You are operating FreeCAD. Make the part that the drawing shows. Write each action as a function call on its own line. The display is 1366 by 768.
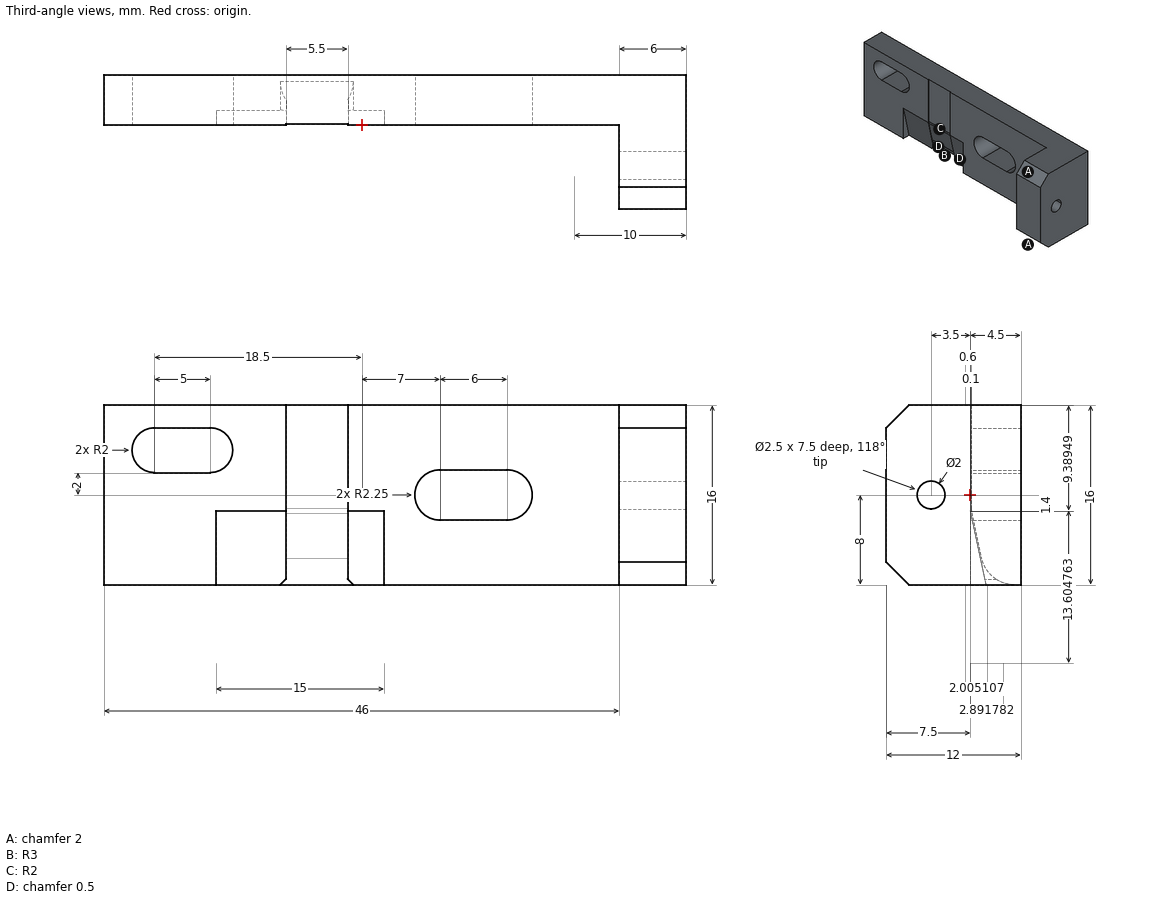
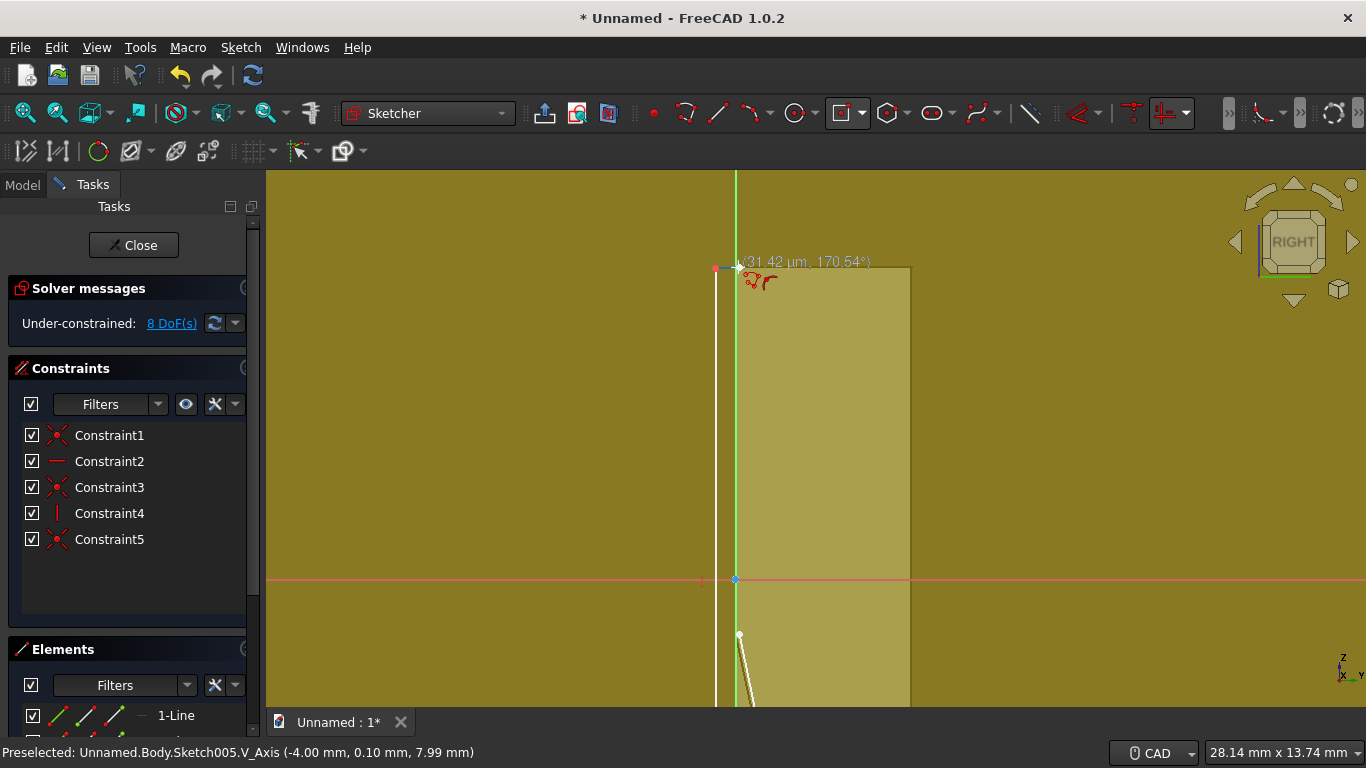
scroll(739, 469, up, 11)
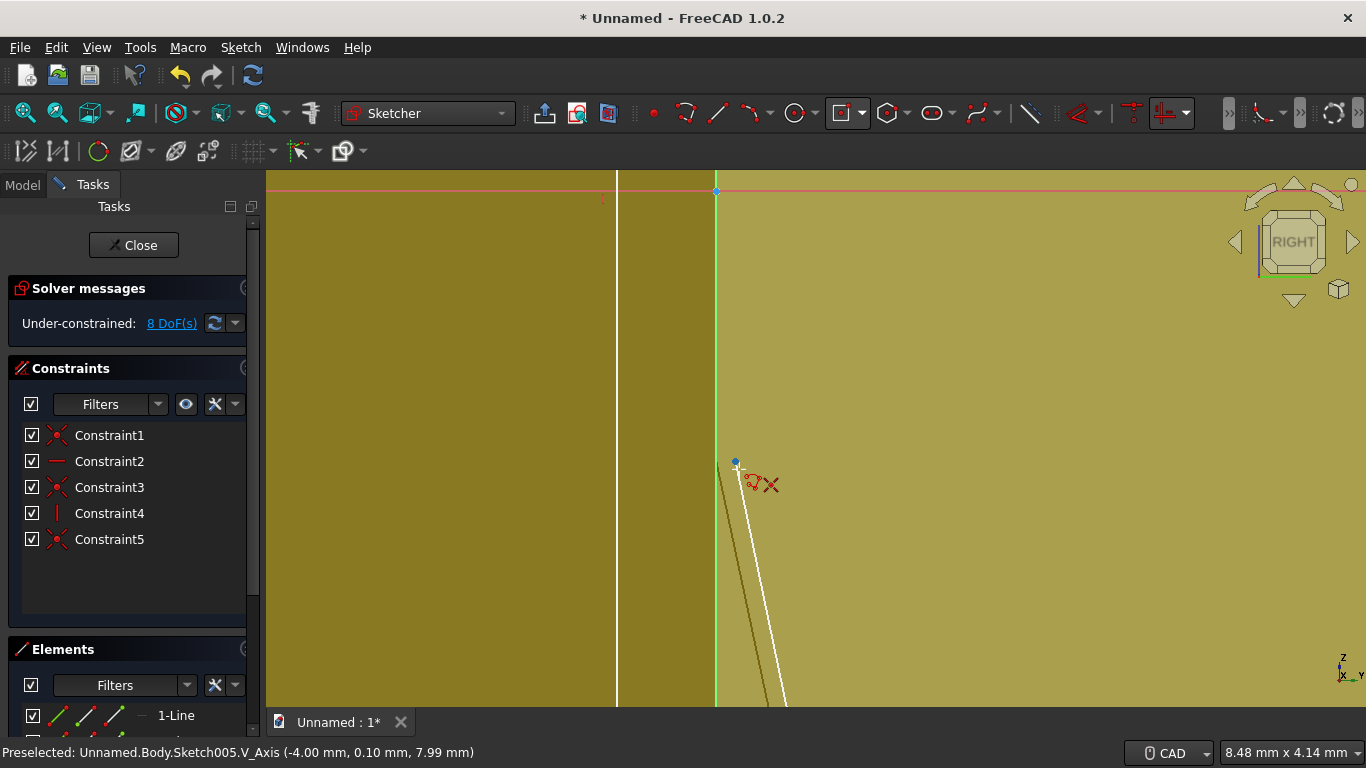
click(735, 461)
key(Escape)
key(Escape)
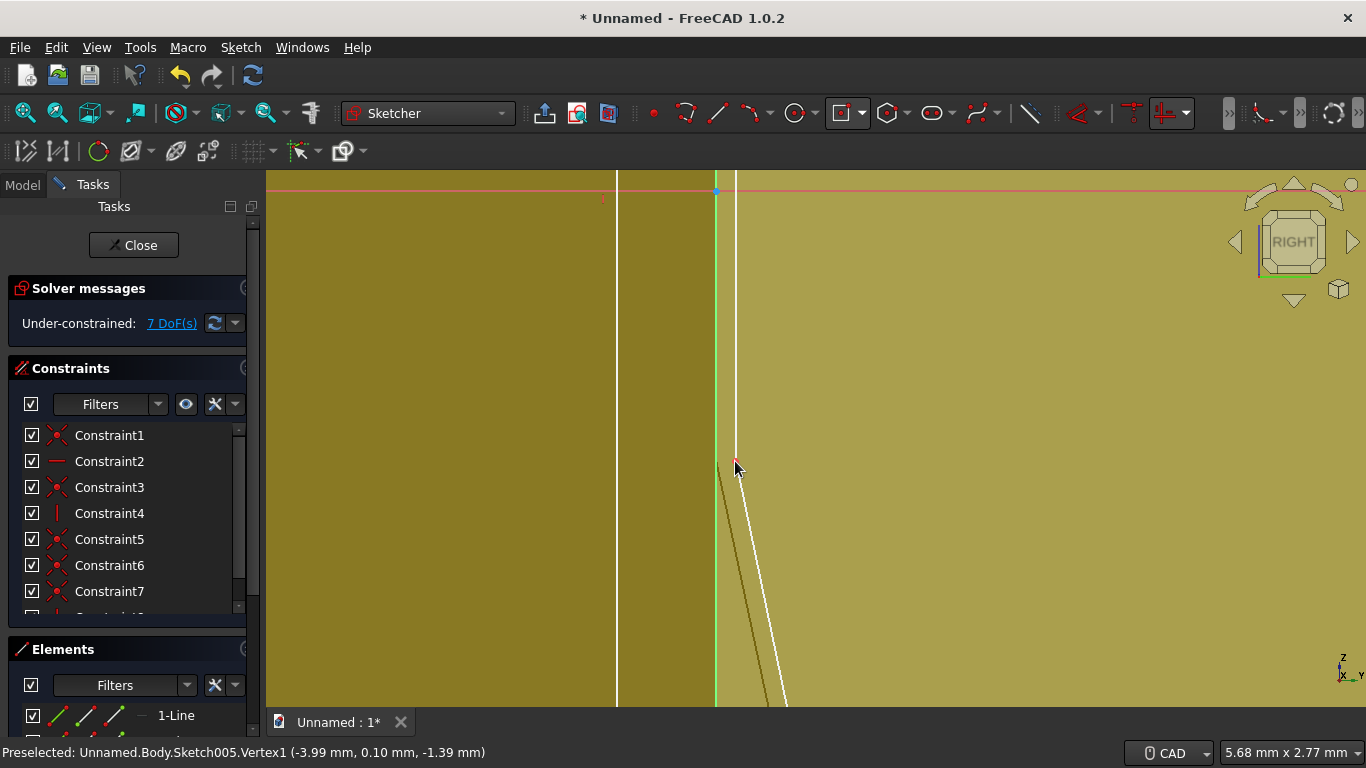
scroll(739, 469, down, 11)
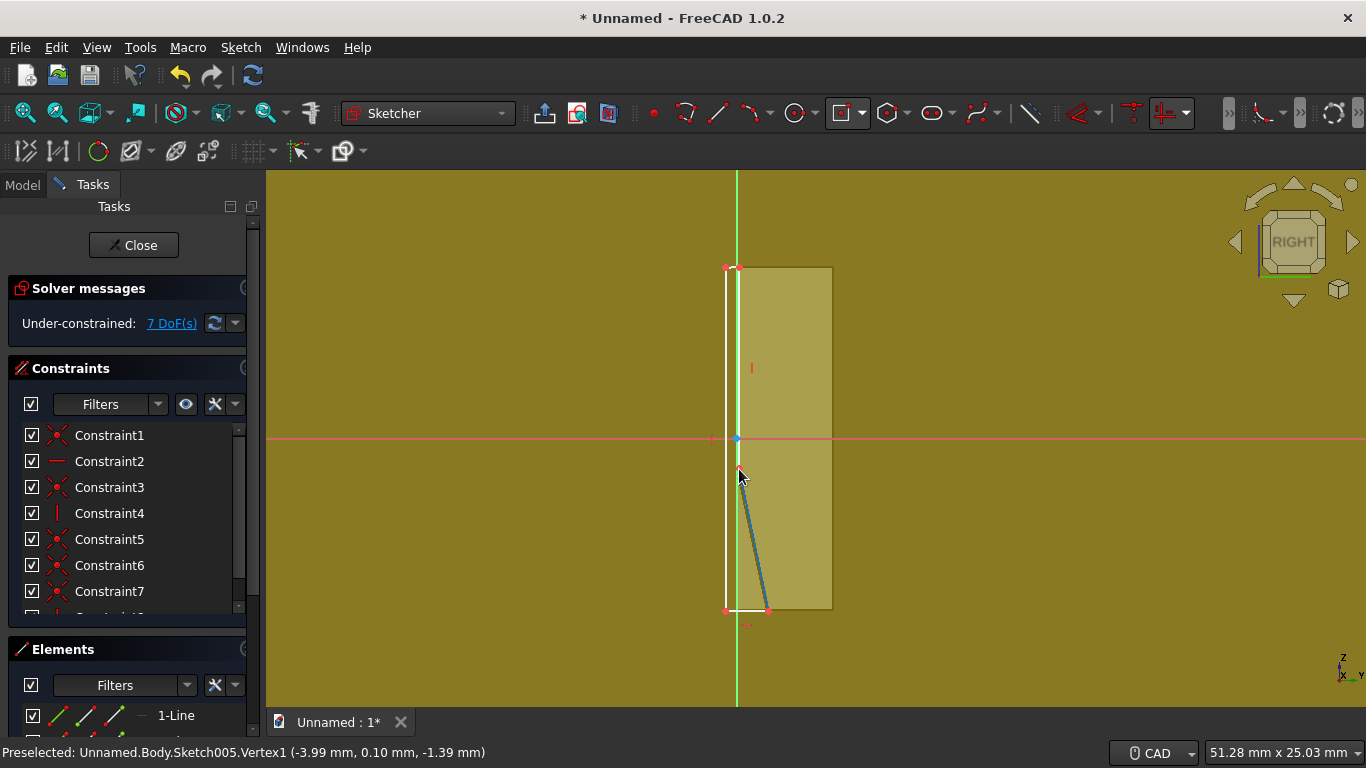
scroll(730, 268, up, 7)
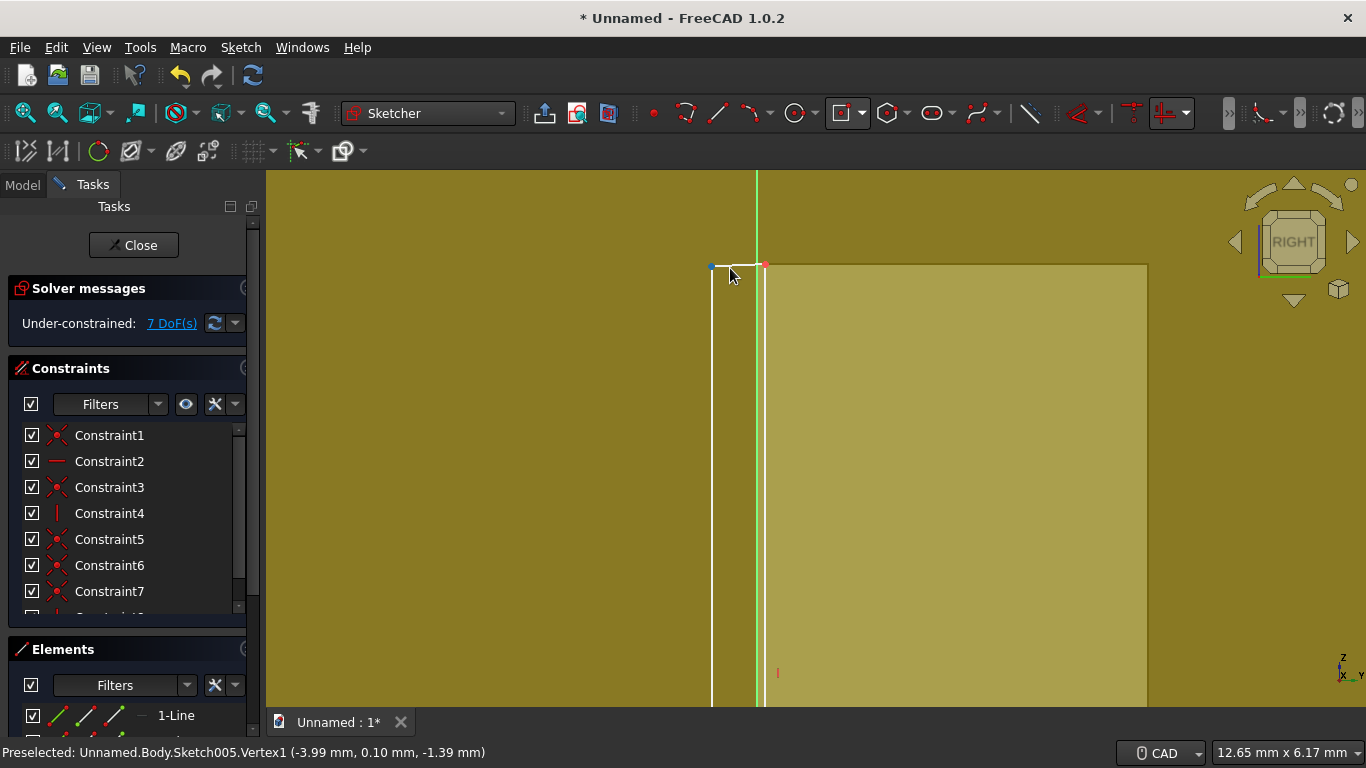
click(728, 266)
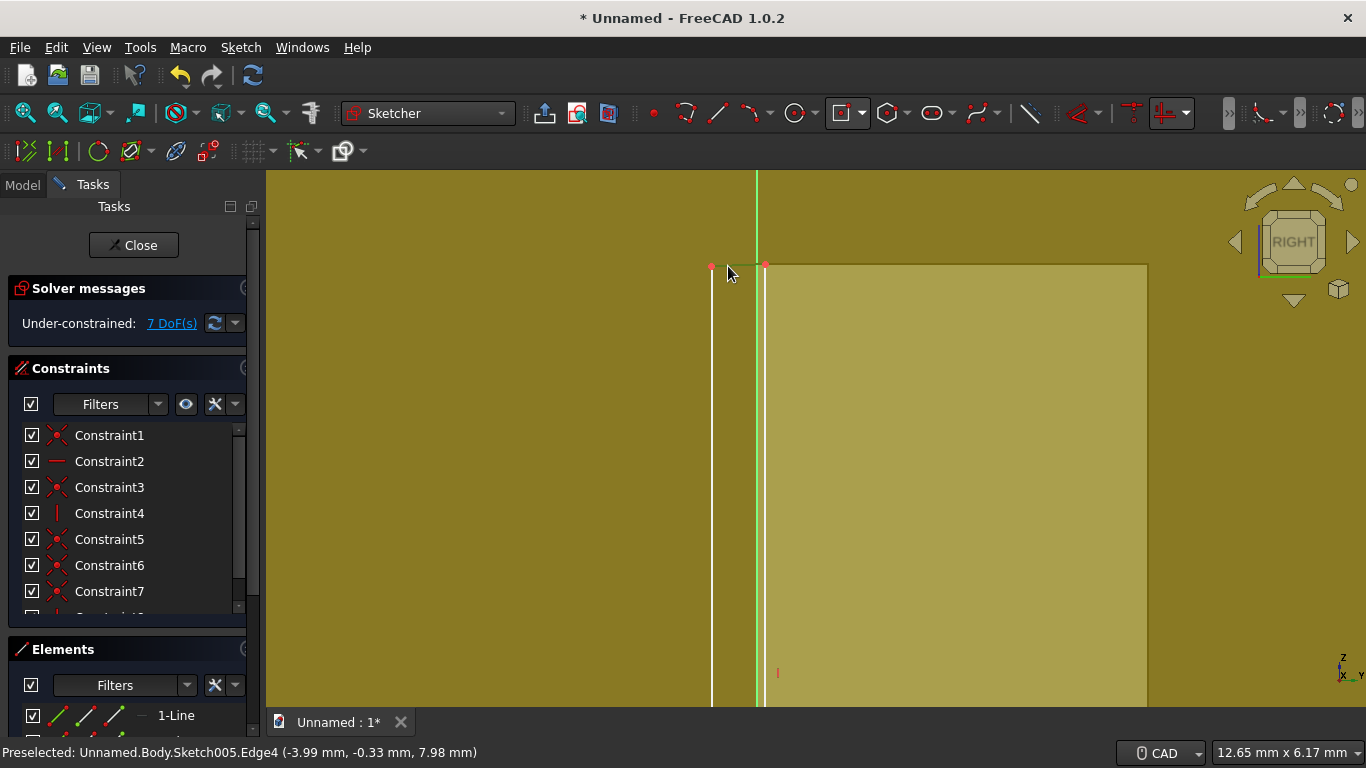
key(h)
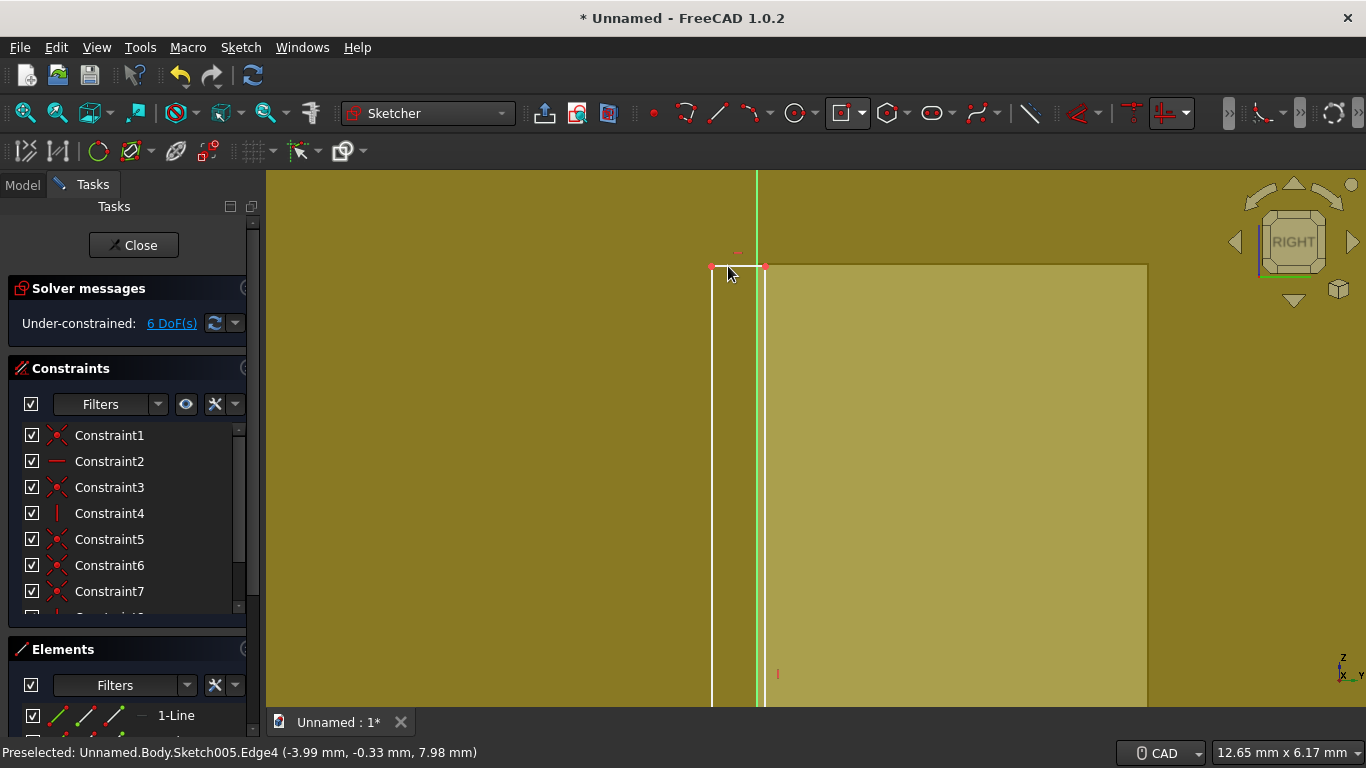
key(d)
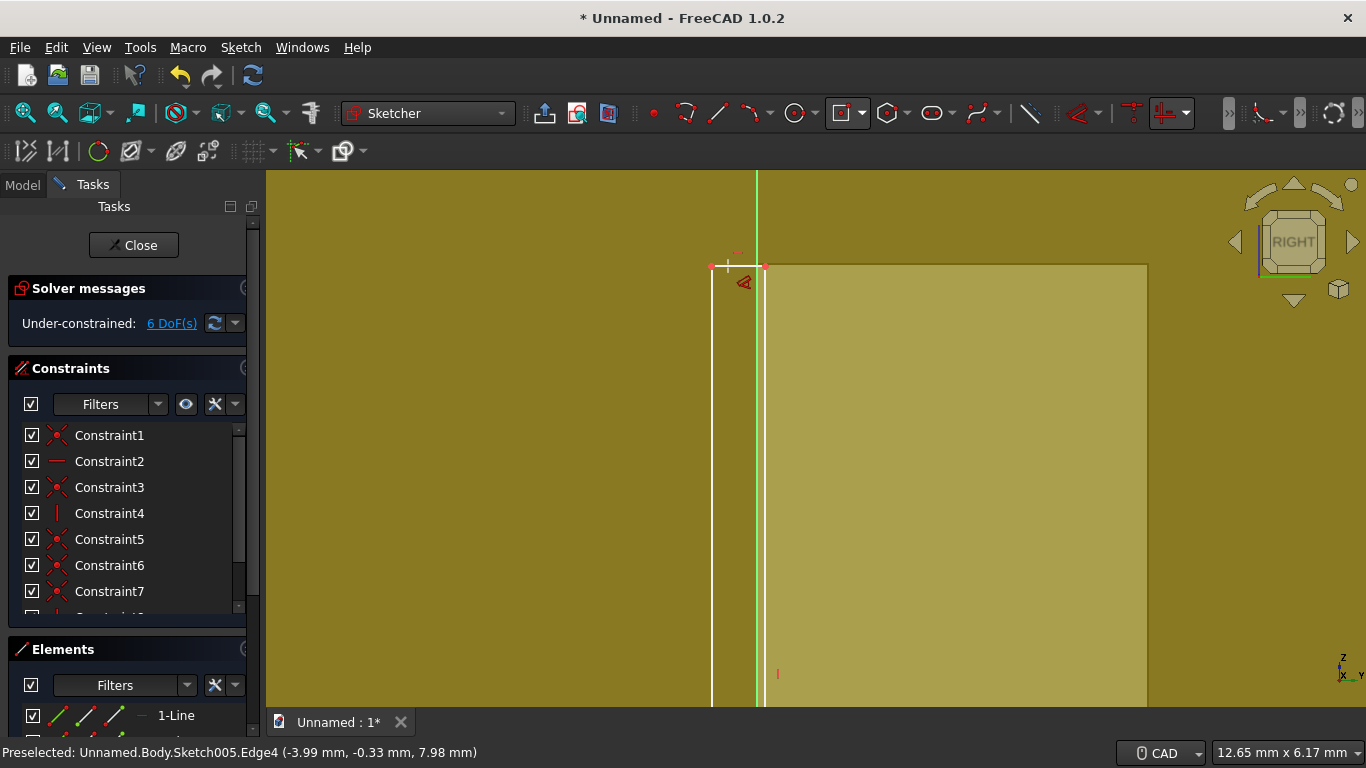
scroll(730, 268, down, 7)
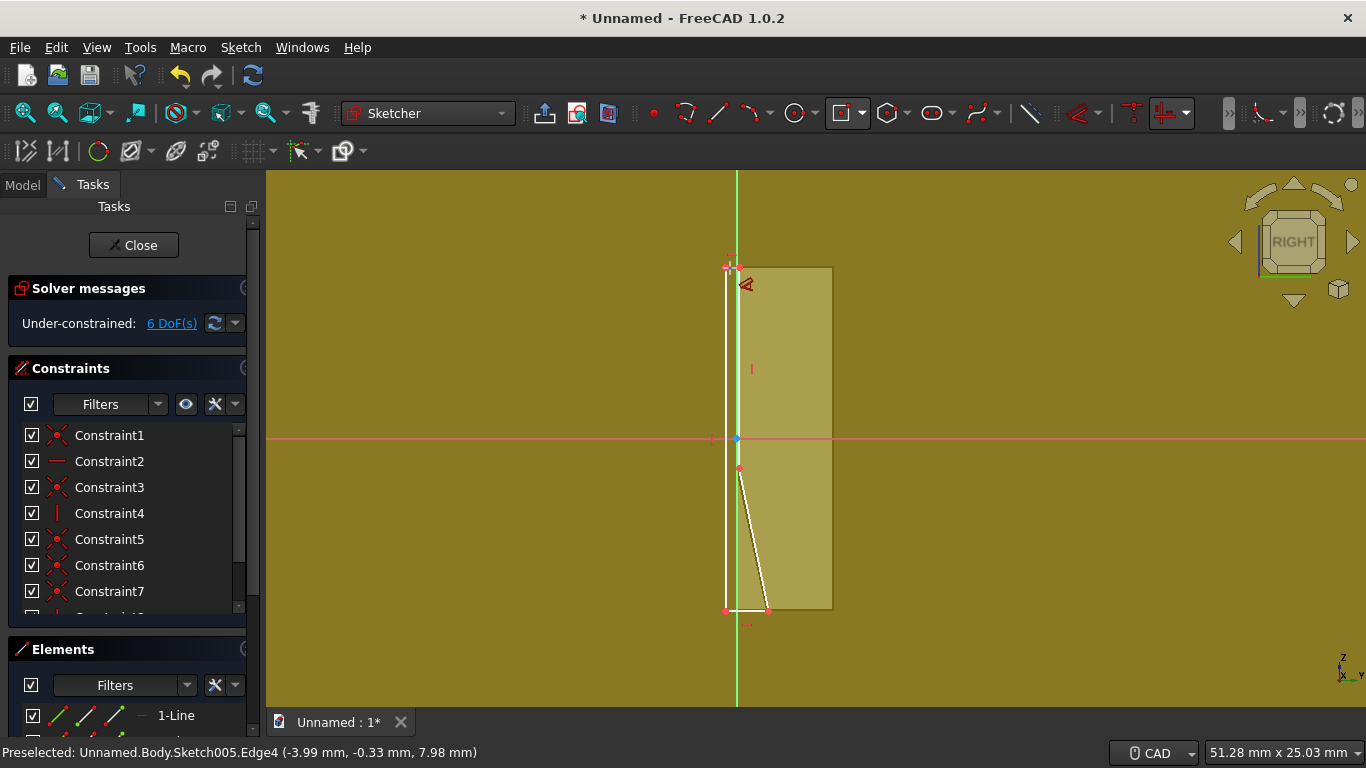
scroll(726, 336, up, 2)